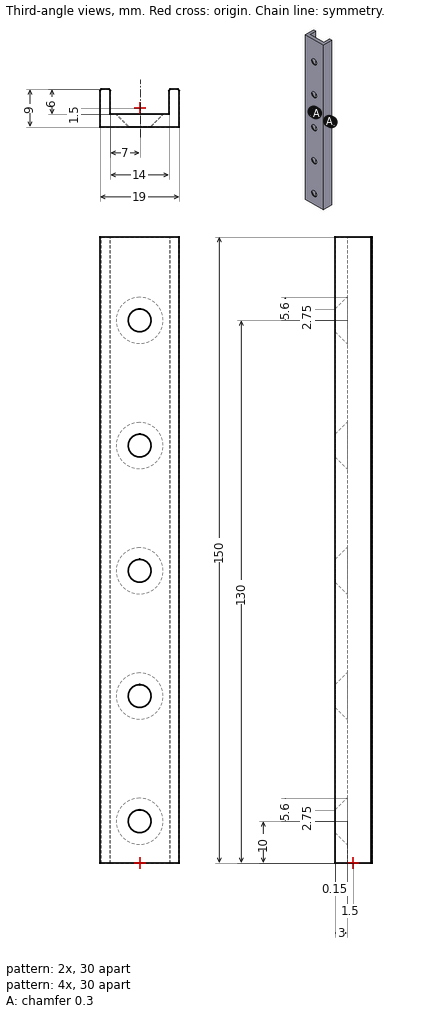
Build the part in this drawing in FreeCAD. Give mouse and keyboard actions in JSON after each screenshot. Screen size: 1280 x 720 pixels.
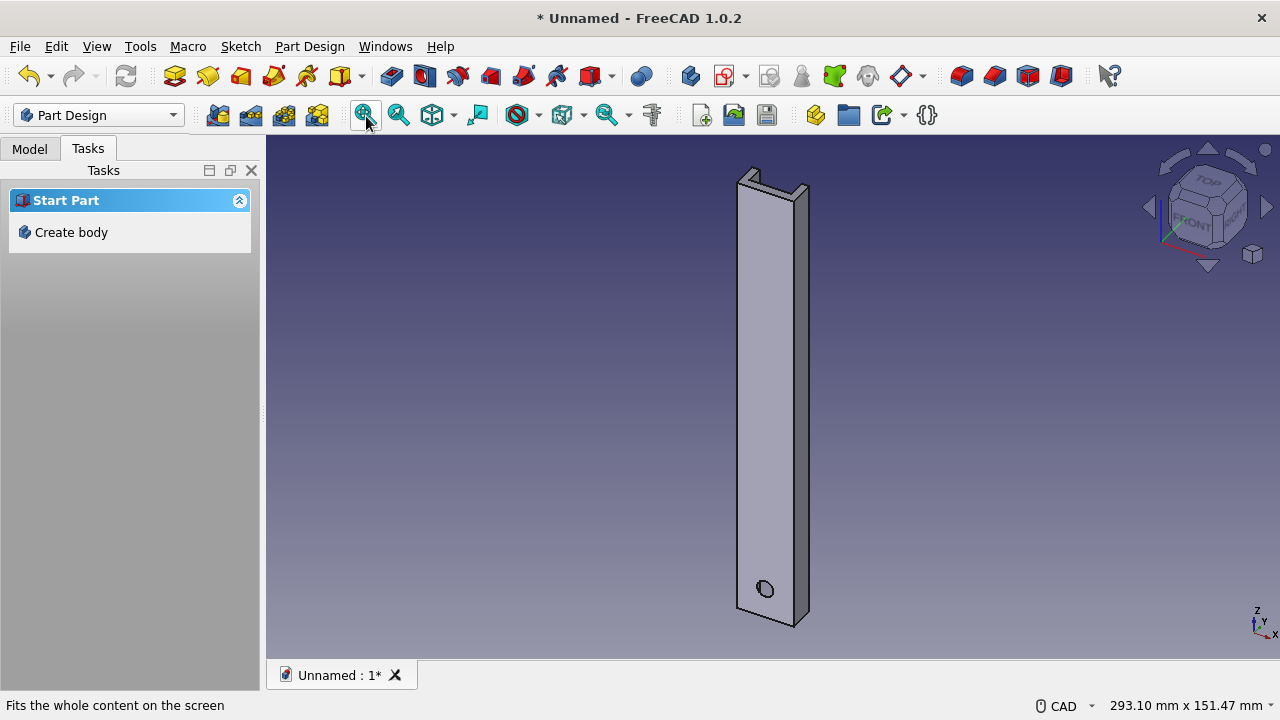
{"action": "left_click", "coordinate": [30, 148]}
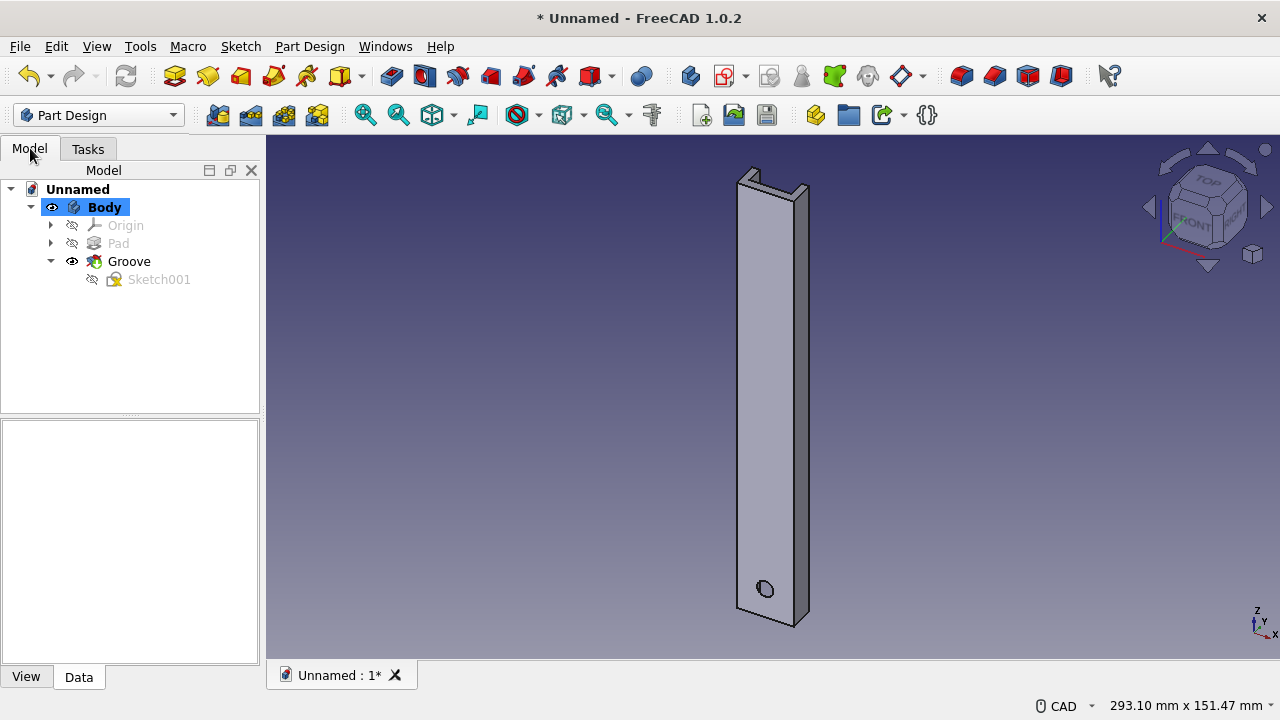
{"action": "left_click", "coordinate": [117, 261]}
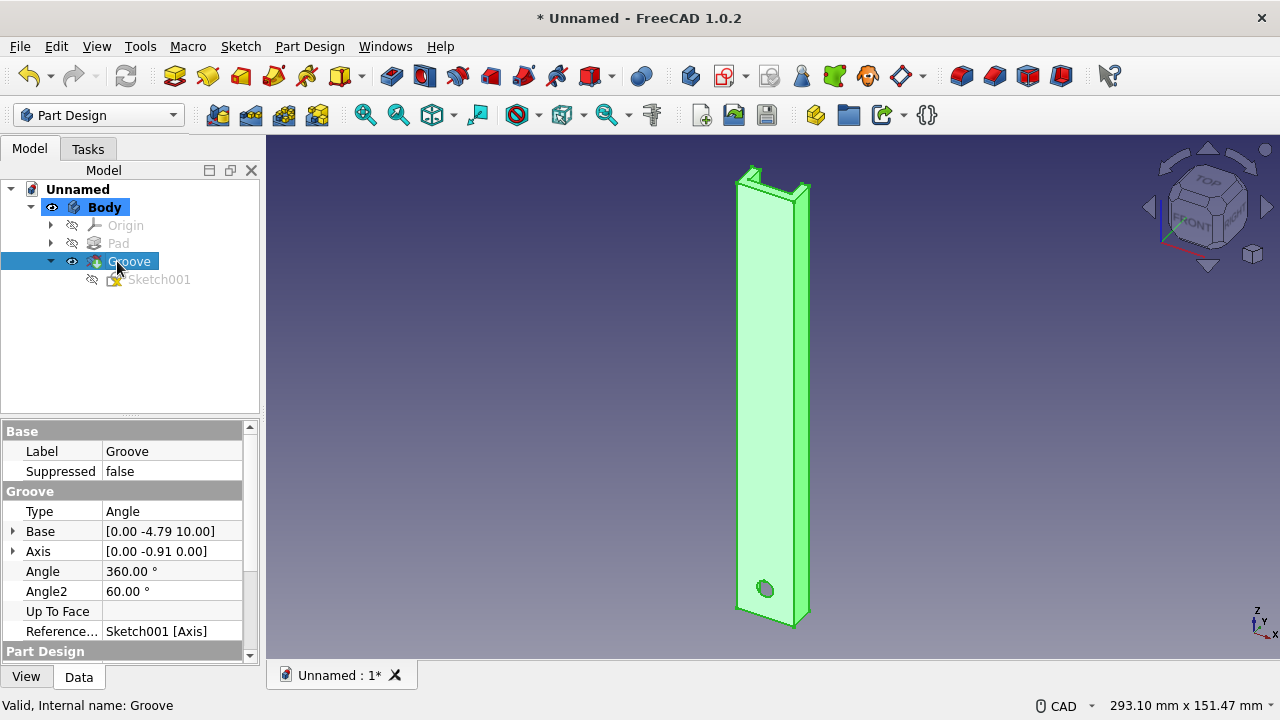
{"action": "left_click", "coordinate": [251, 116]}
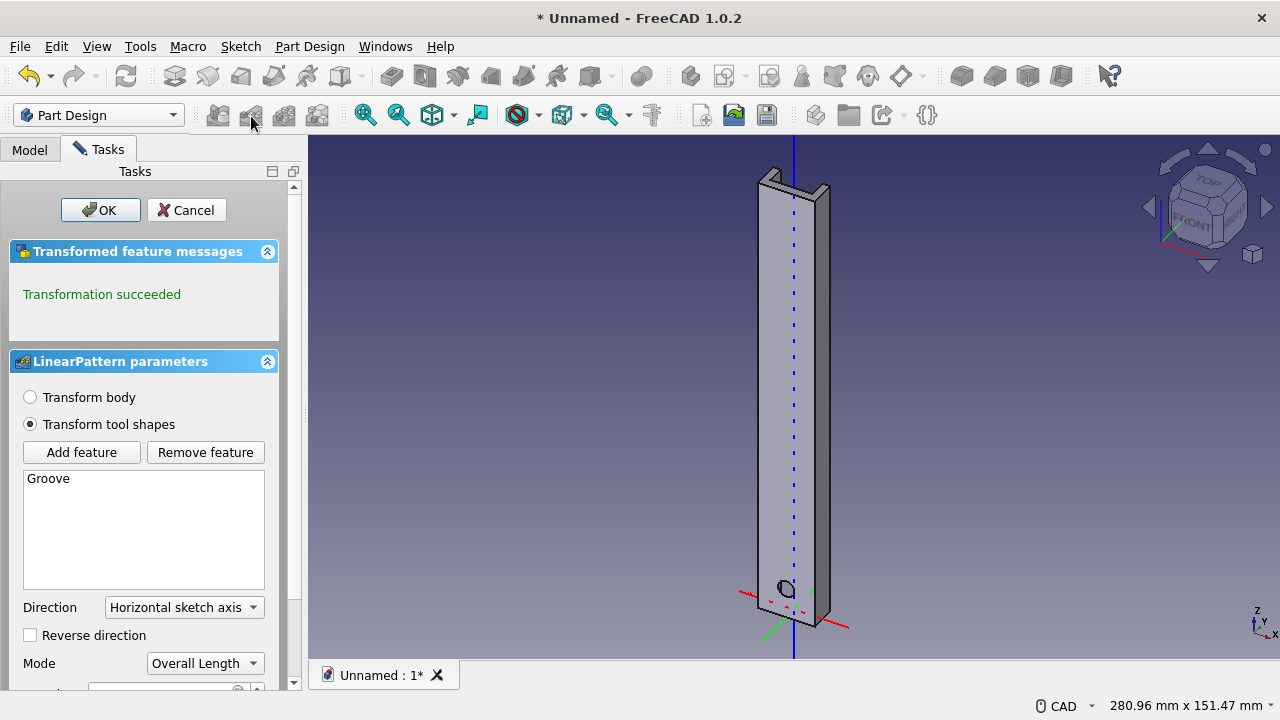
{"action": "left_click", "coordinate": [185, 608]}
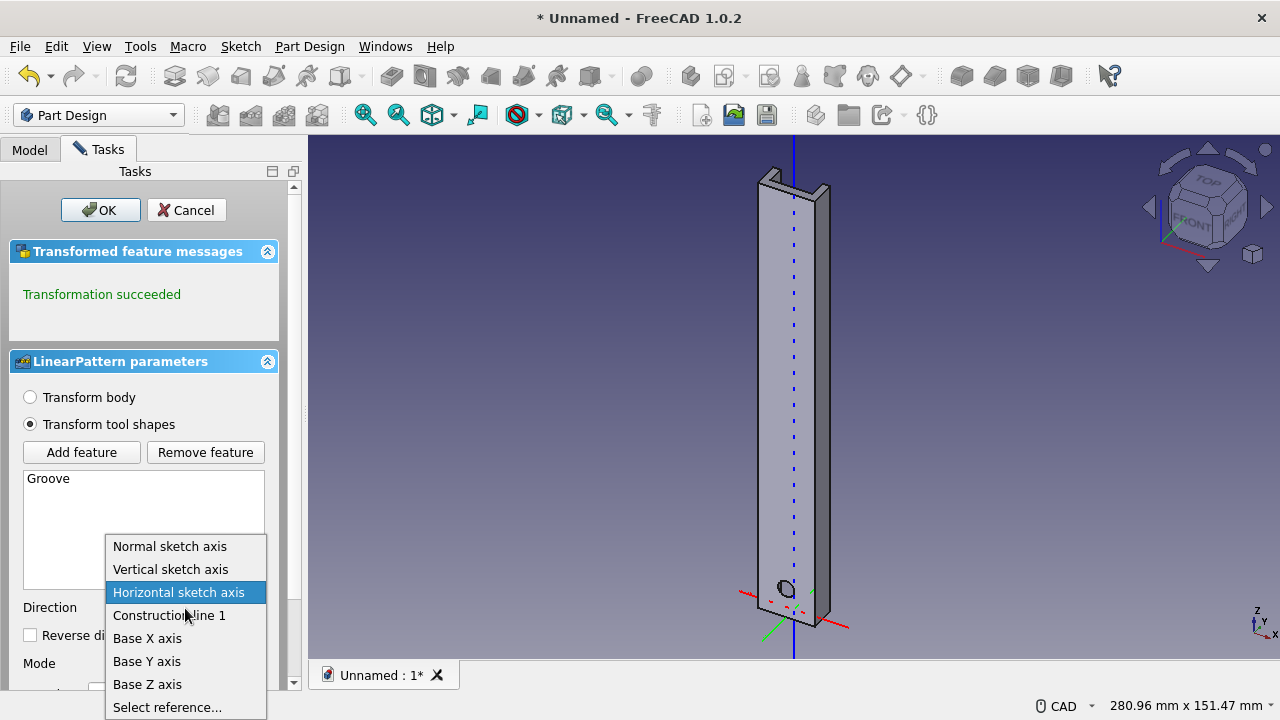
{"action": "left_click", "coordinate": [184, 684]}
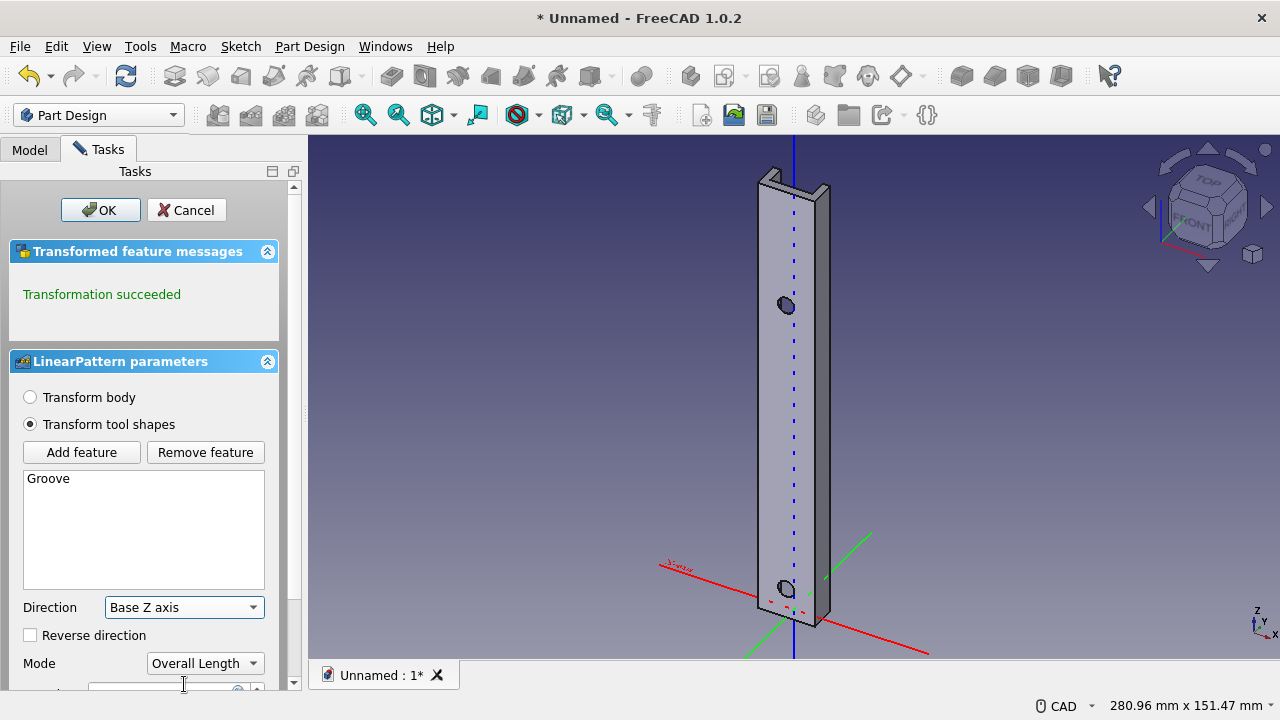
{"action": "left_click", "coordinate": [206, 664]}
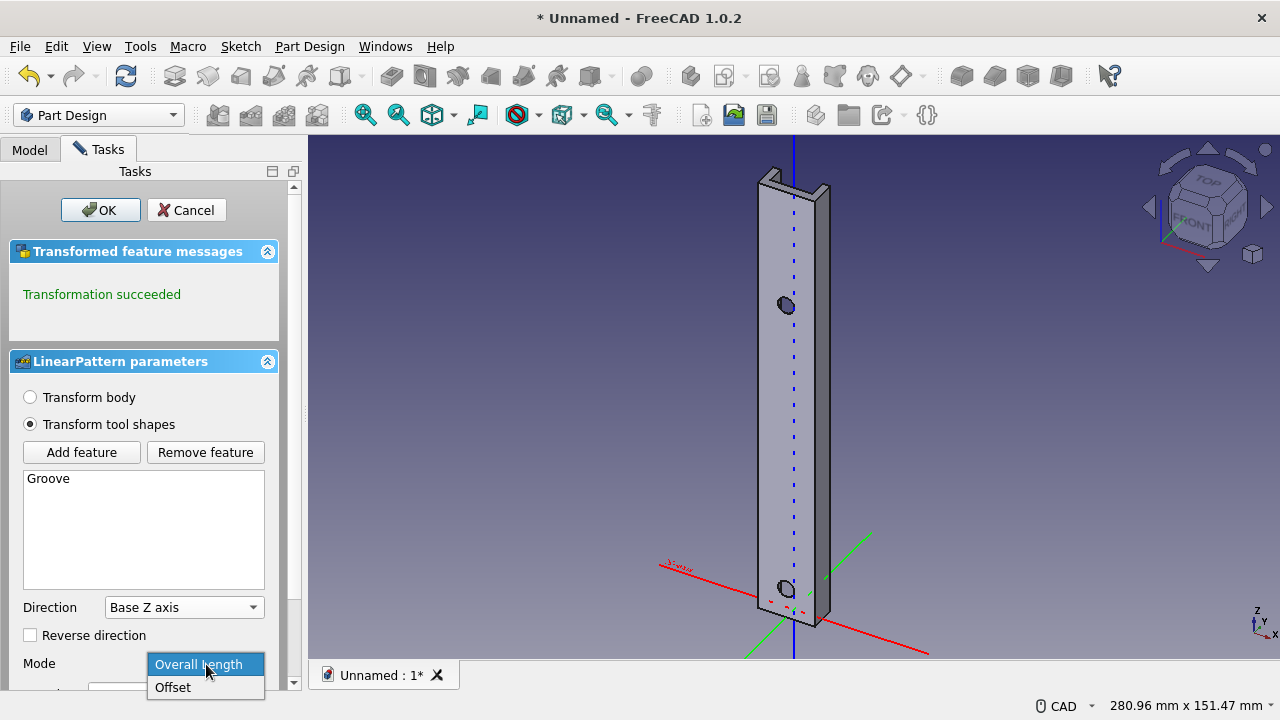
{"action": "left_click", "coordinate": [204, 688]}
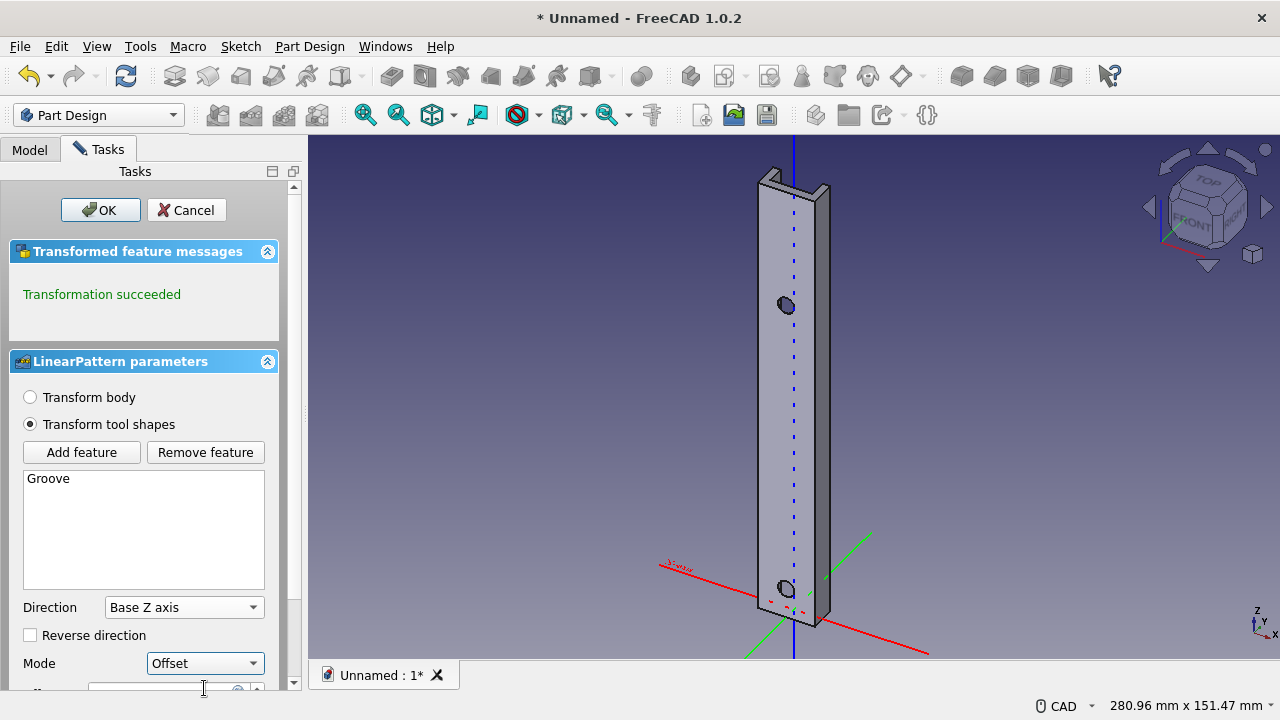
{"action": "scroll", "coordinate": [294, 436], "scroll_direction": "down", "scroll_amount": 2}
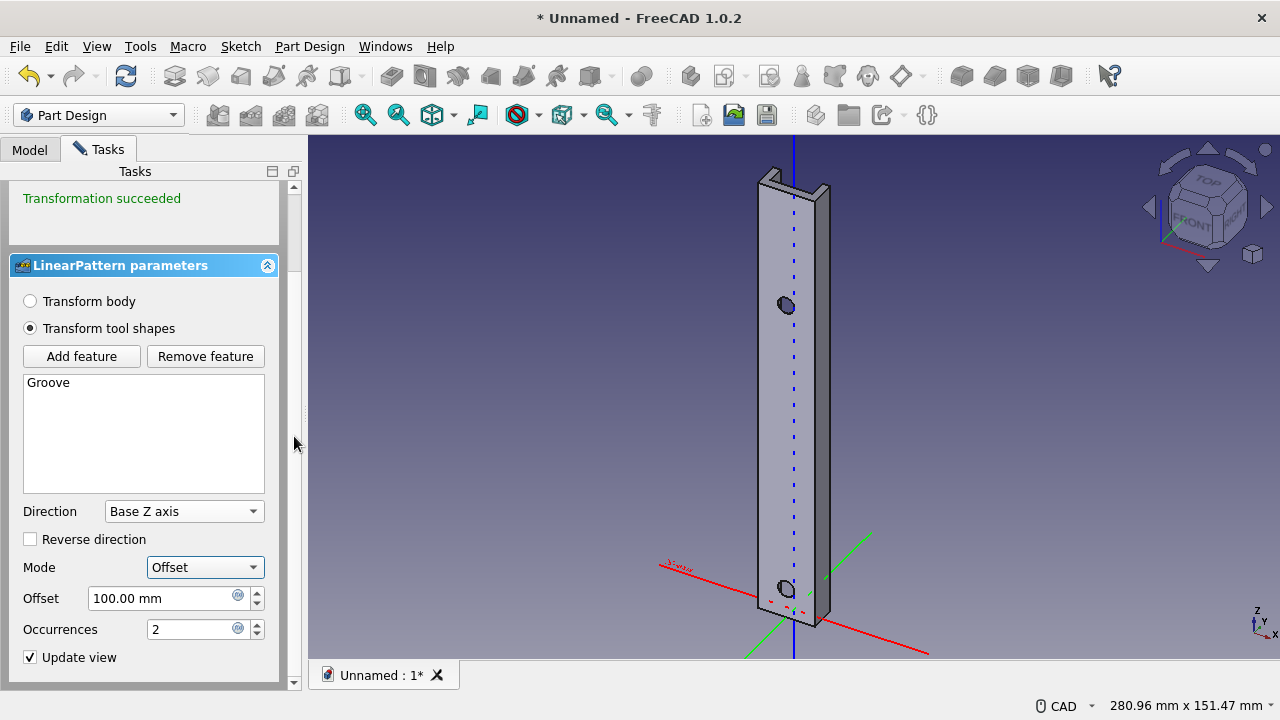
{"action": "triple_click", "coordinate": [170, 598]}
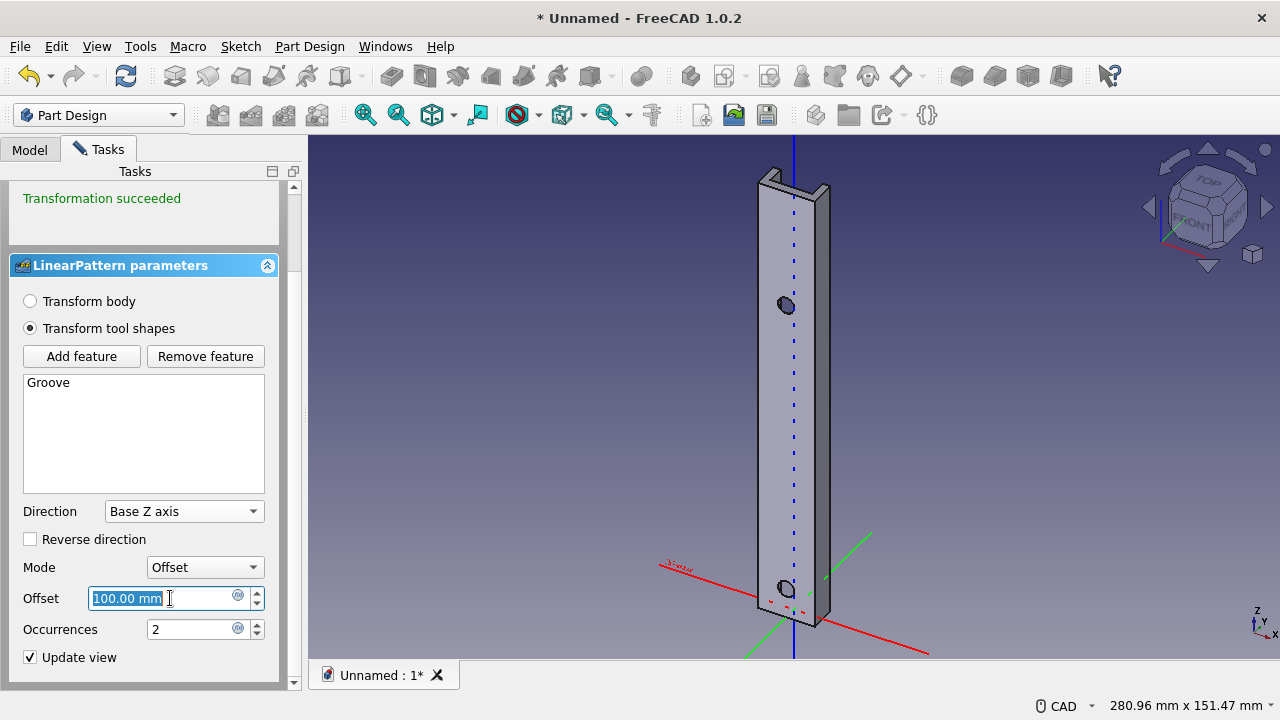
{"action": "type", "text": "30"}
{"action": "key", "text": "Tab"}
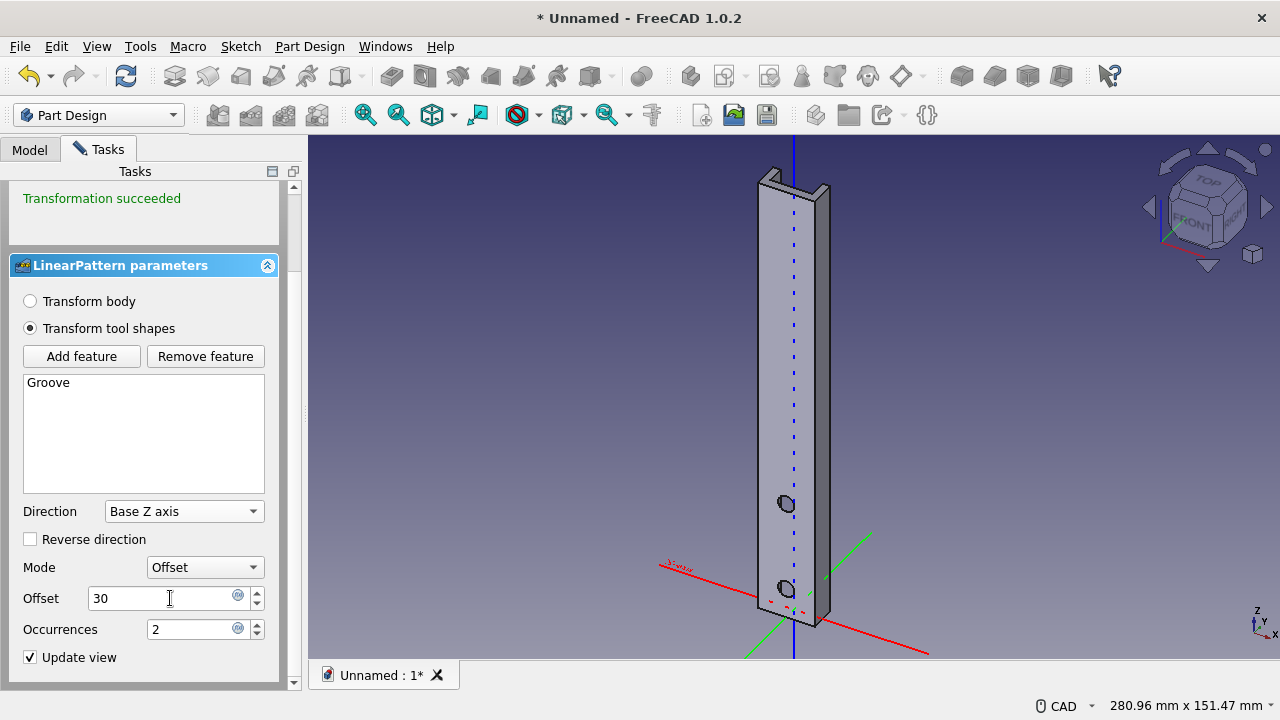
{"action": "triple_click", "coordinate": [199, 630]}